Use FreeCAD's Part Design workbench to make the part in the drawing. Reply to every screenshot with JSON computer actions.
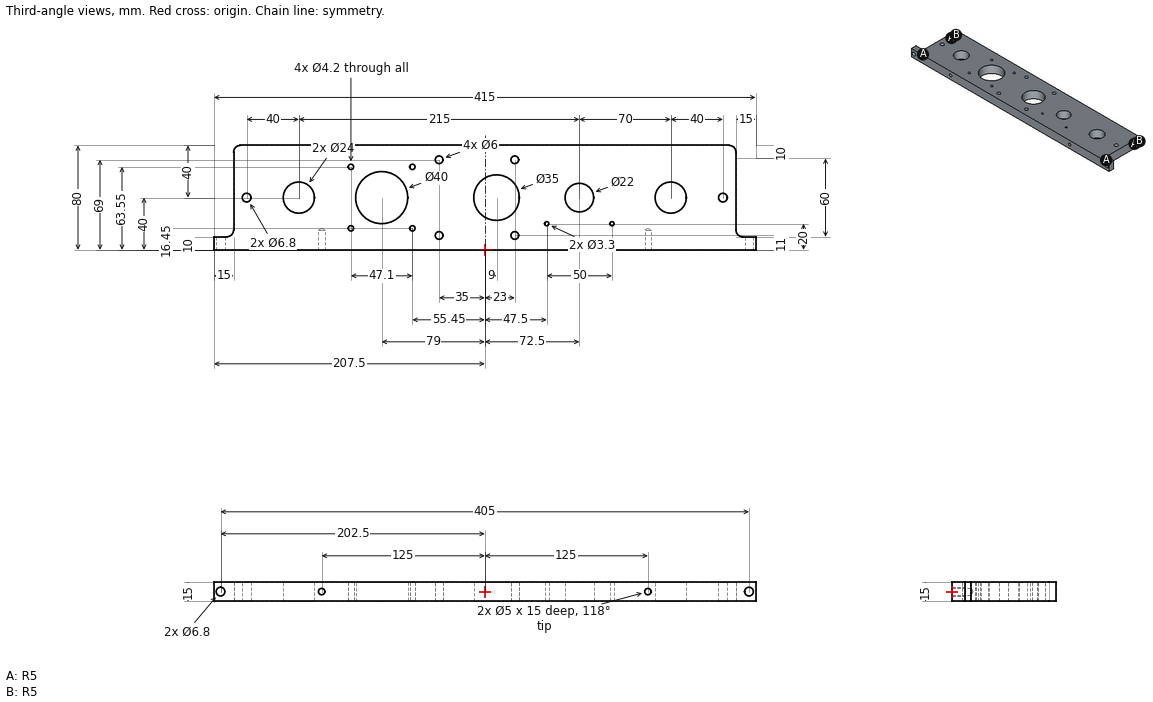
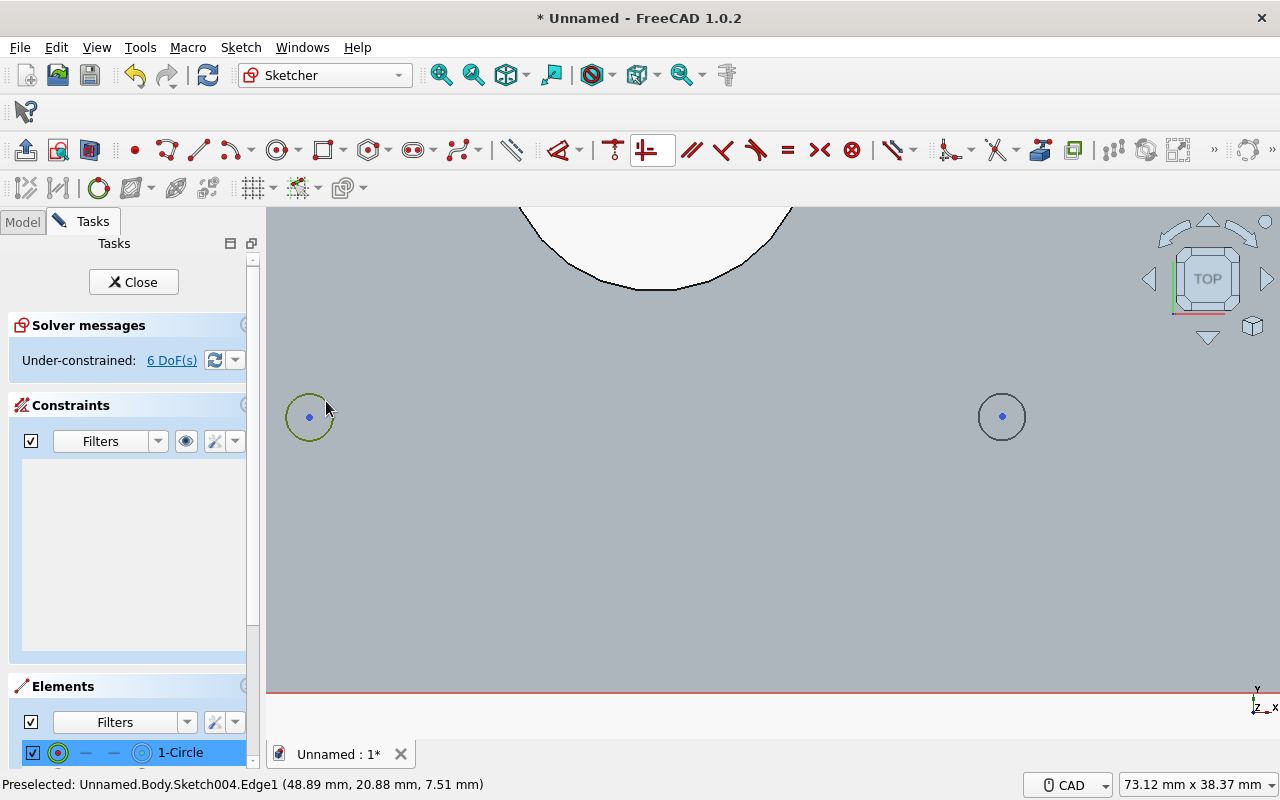
{"action": "left_click", "coordinate": [1018, 400]}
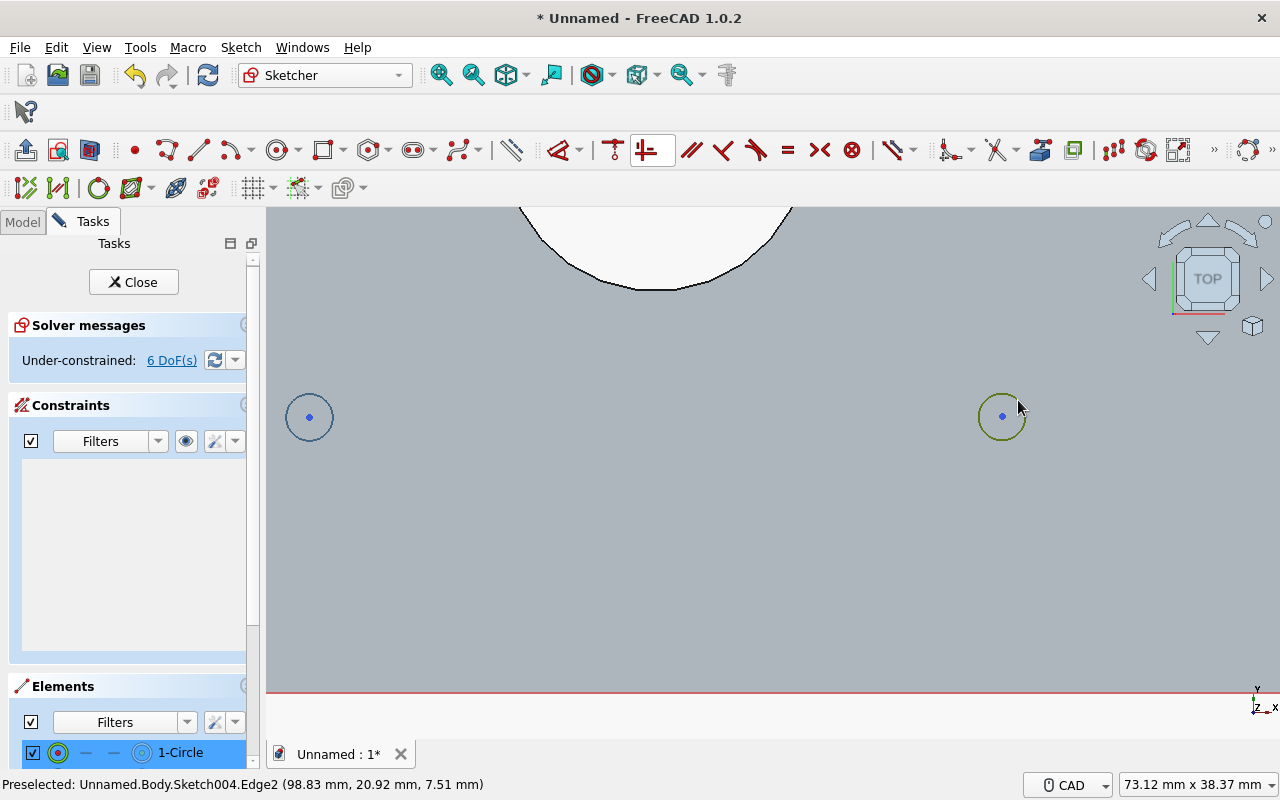
{"action": "left_click", "coordinate": [788, 150]}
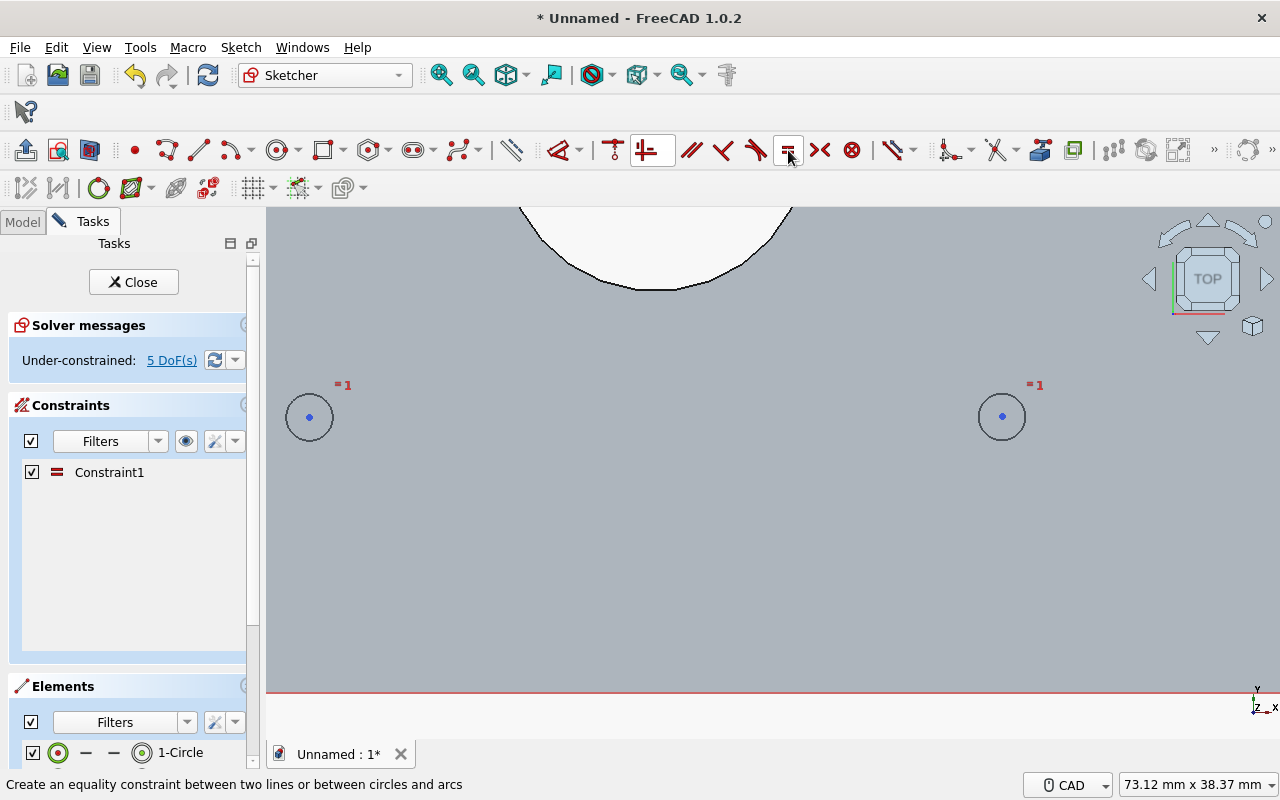
{"action": "left_click", "coordinate": [309, 417]}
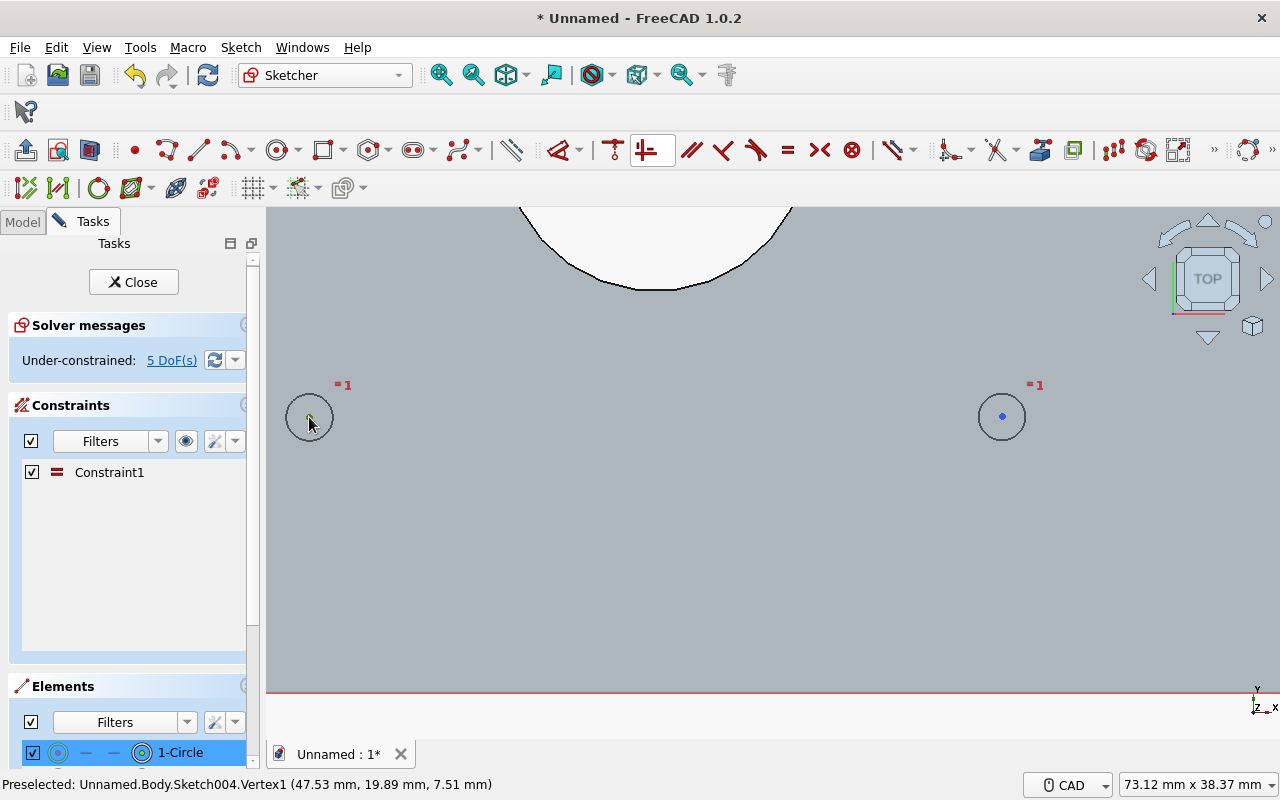
{"action": "left_click", "coordinate": [1002, 417]}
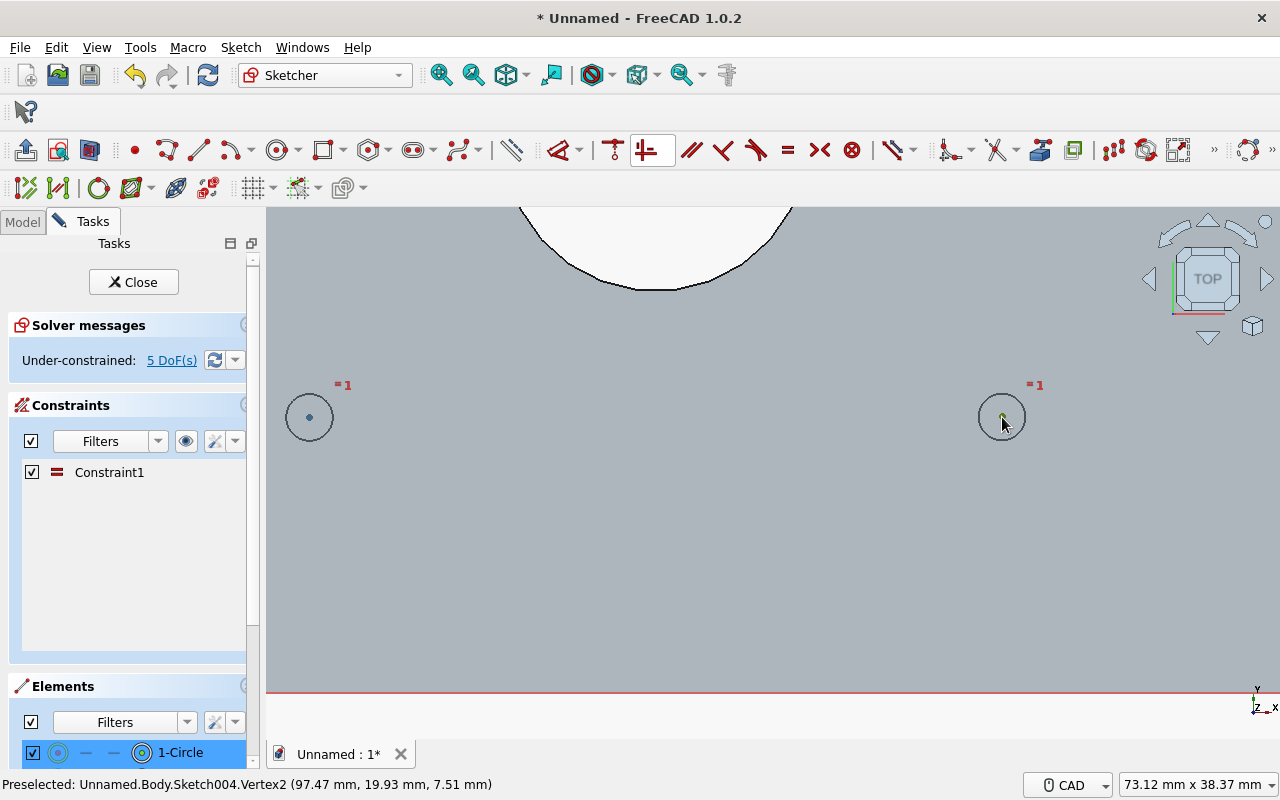
{"action": "key", "text": "h"}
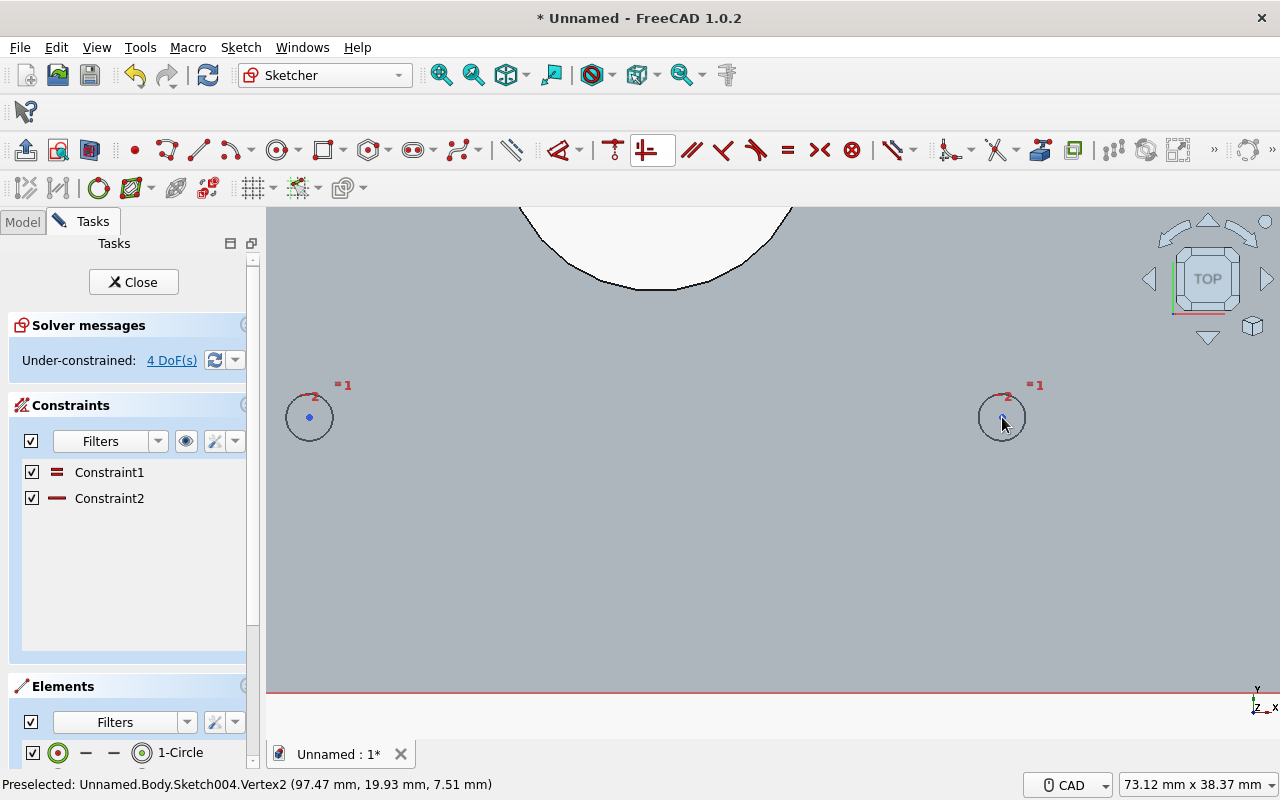
{"action": "left_click", "coordinate": [558, 150]}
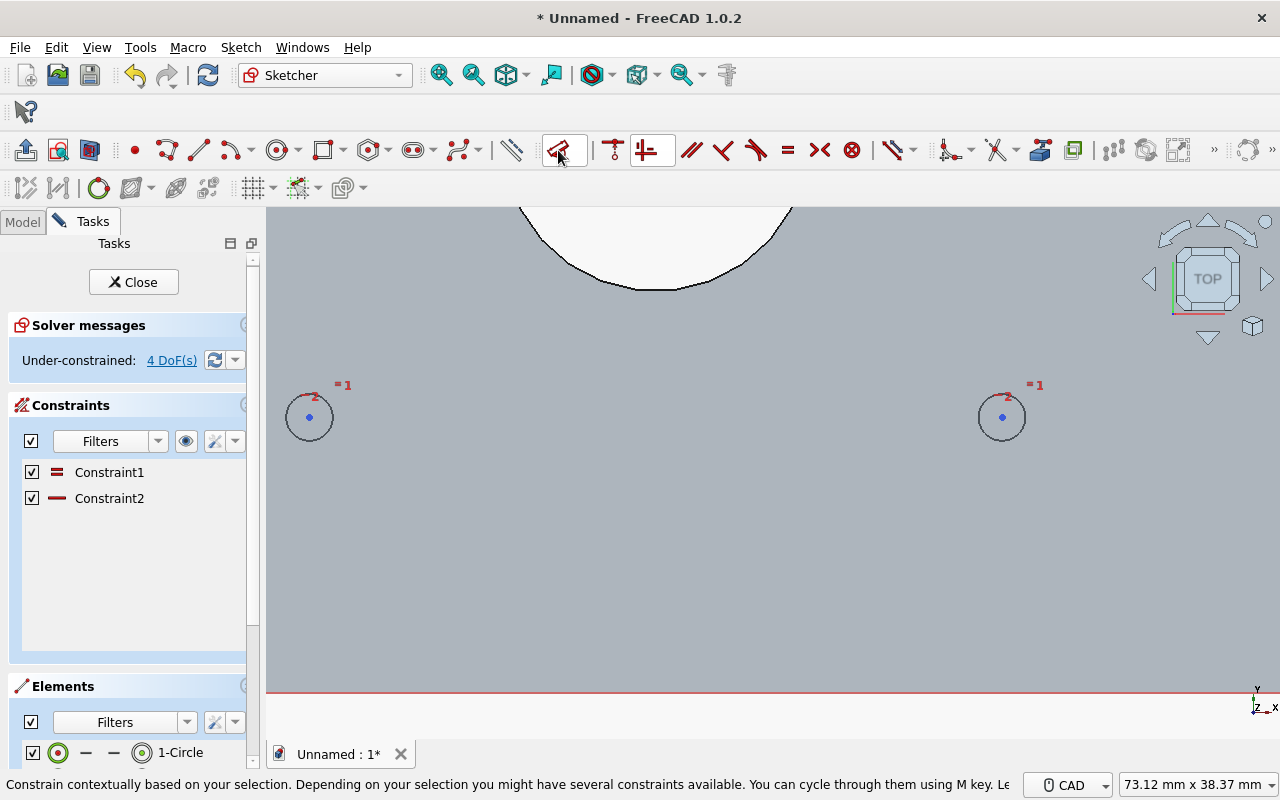
{"action": "left_click", "coordinate": [326, 401]}
{"action": "left_click", "coordinate": [349, 378]}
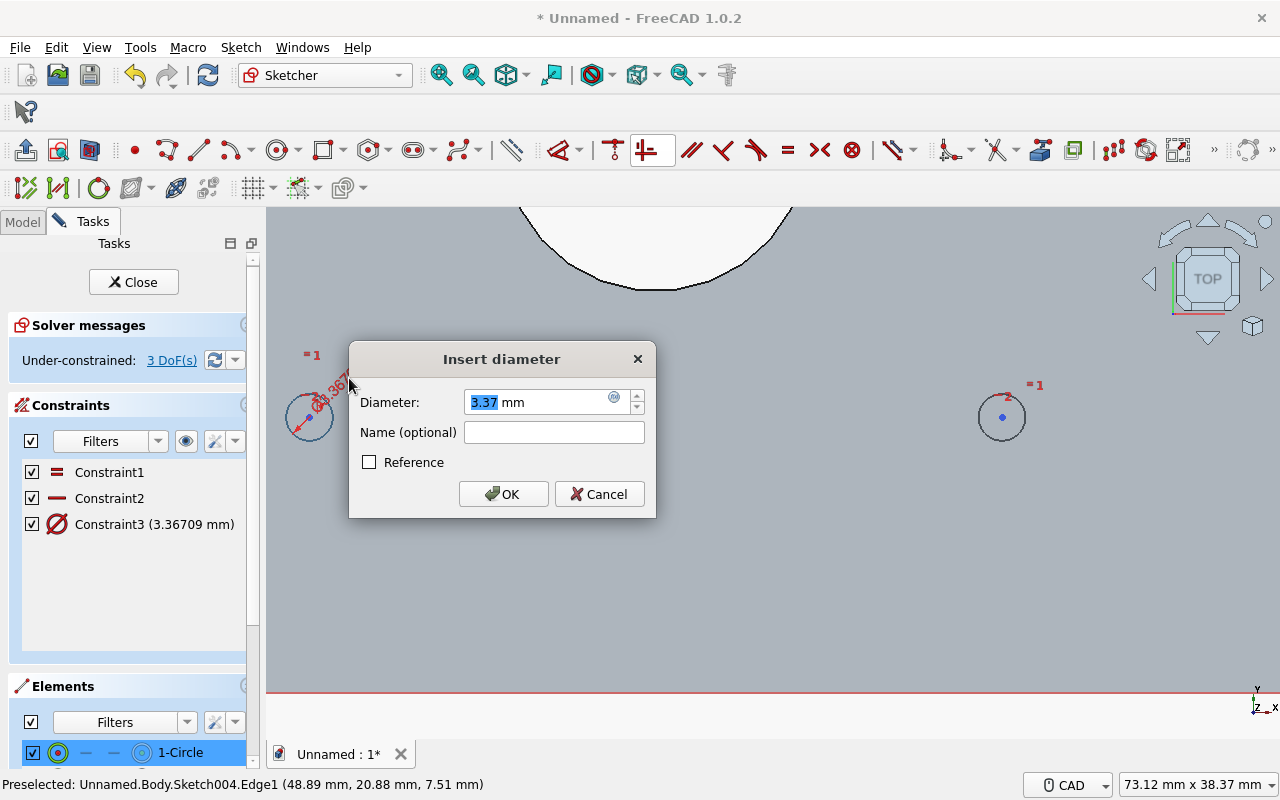
{"action": "type", "text": "3.3"}
{"action": "key", "text": "Return"}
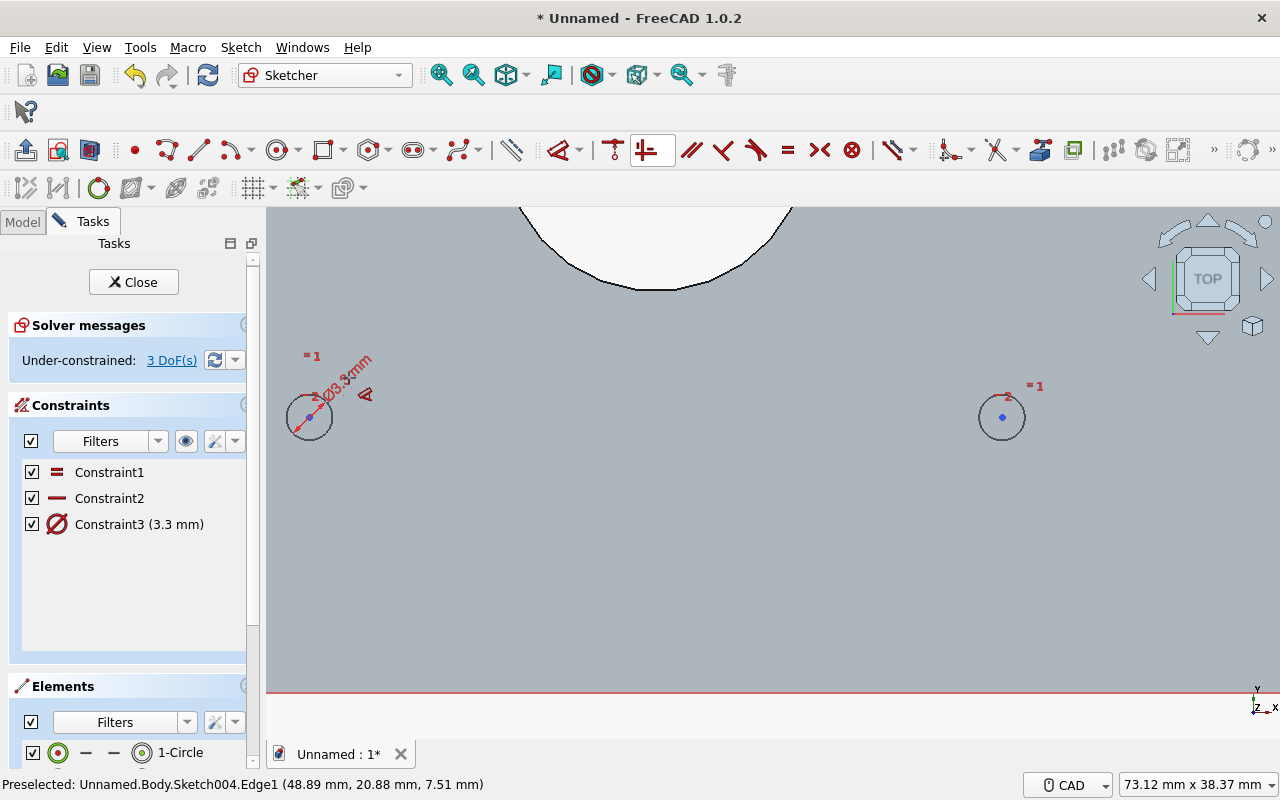
{"action": "left_click", "coordinate": [309, 417]}
{"action": "left_click", "coordinate": [343, 555]}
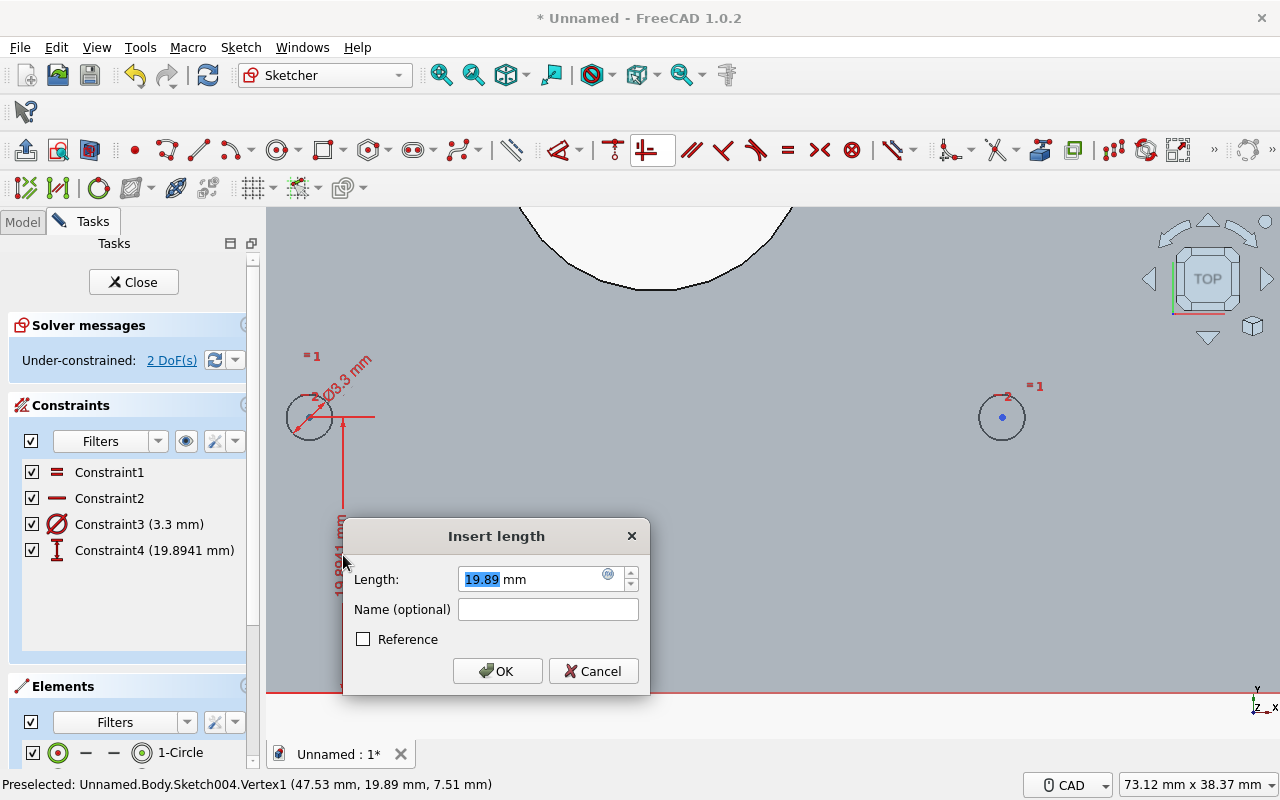
{"action": "type", "text": "20"}
{"action": "key", "text": "Return"}